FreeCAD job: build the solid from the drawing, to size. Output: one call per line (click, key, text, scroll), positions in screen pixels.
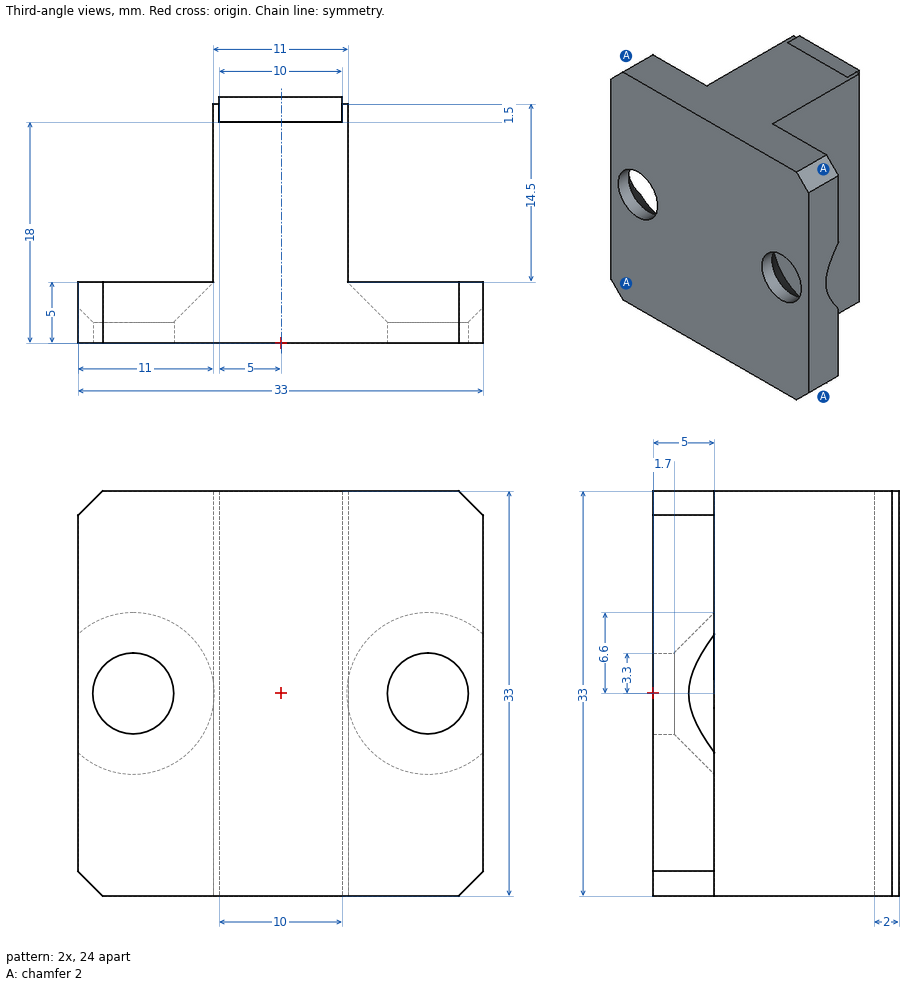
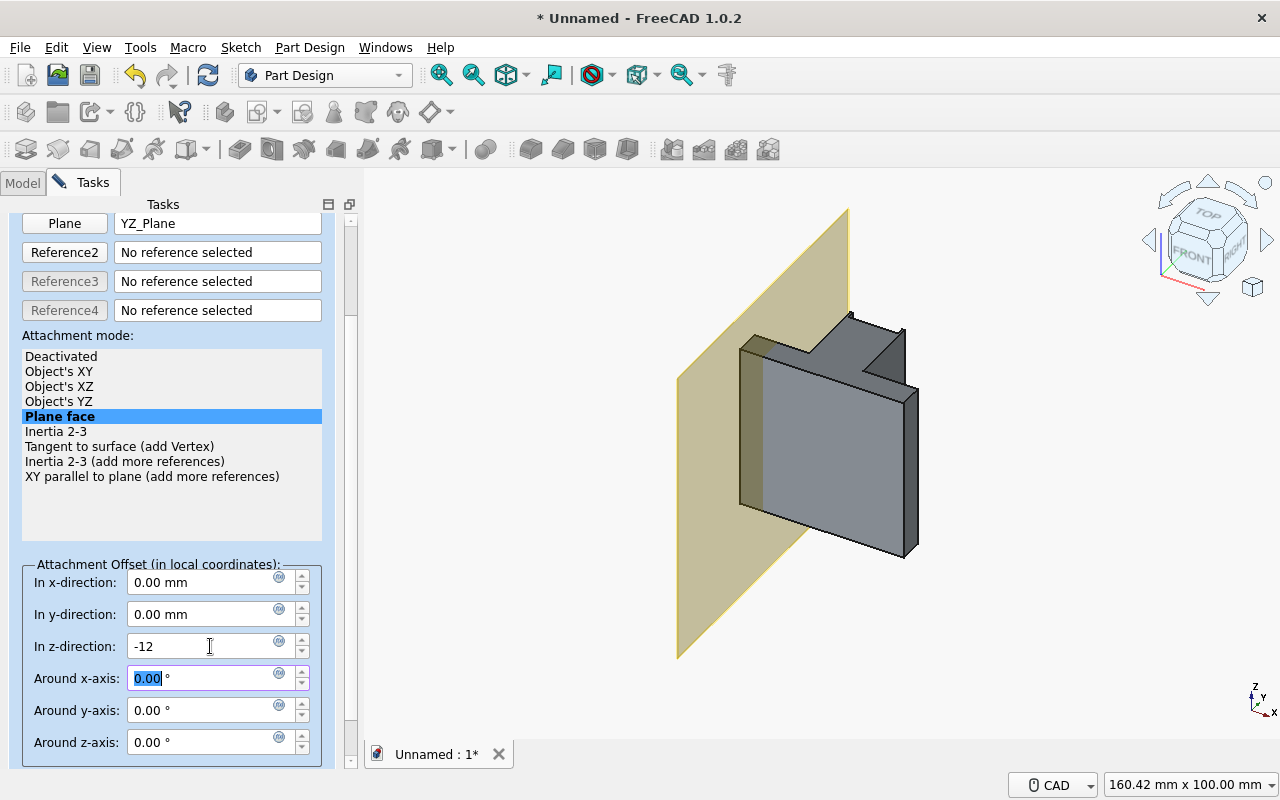
scroll(351, 491, up, 3)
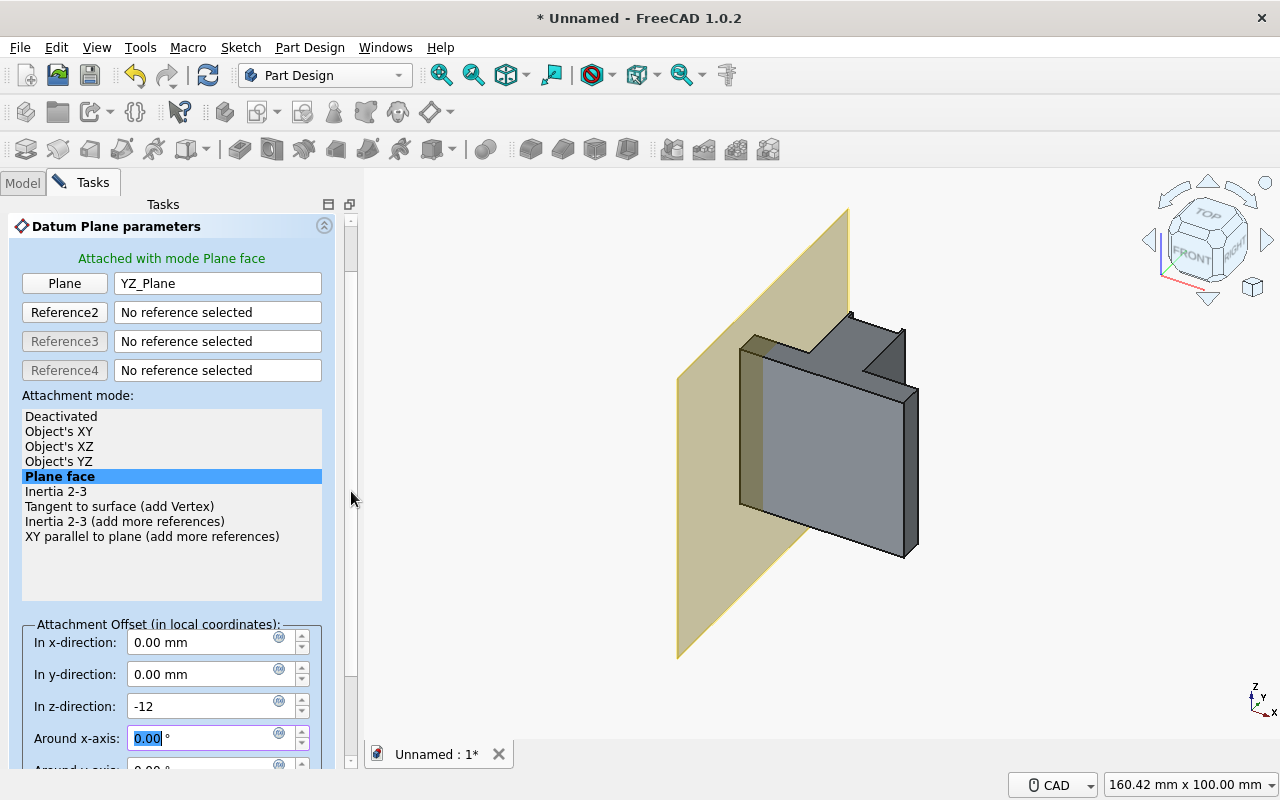
click(124, 243)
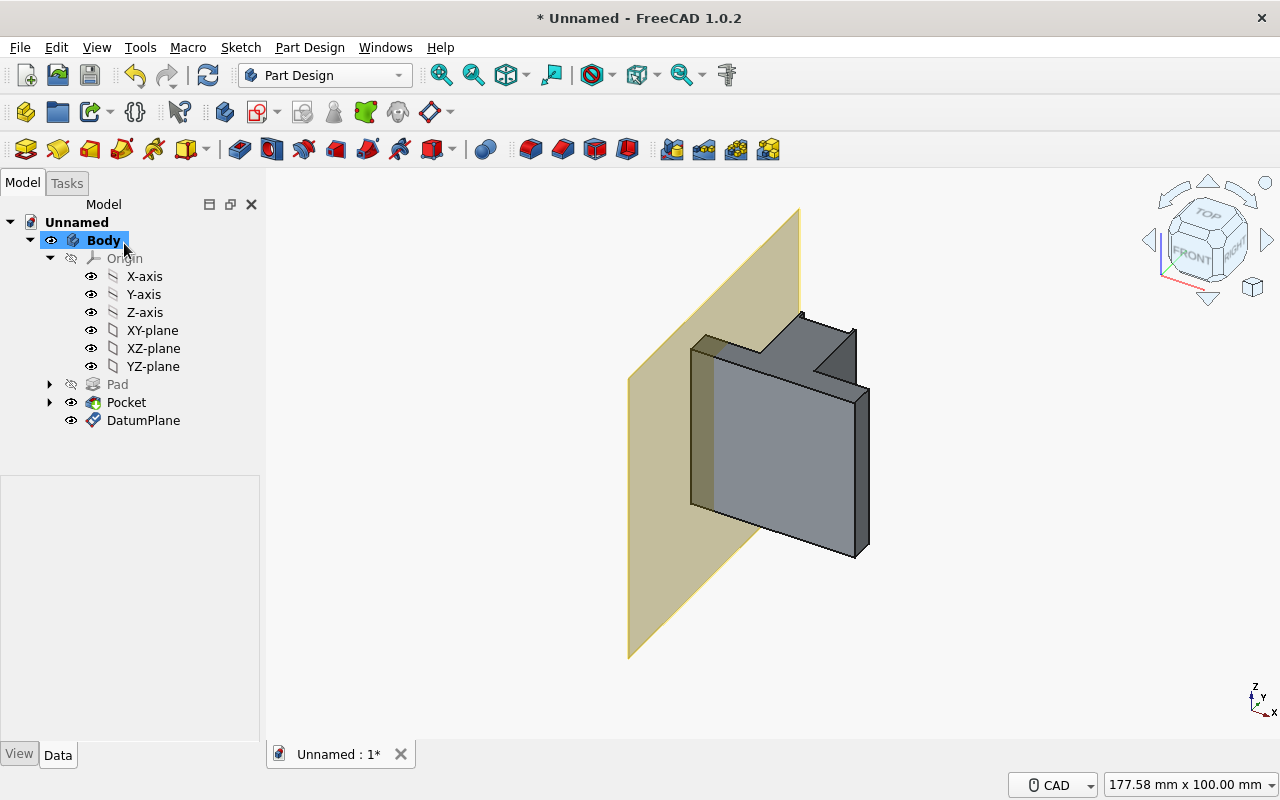
click(116, 420)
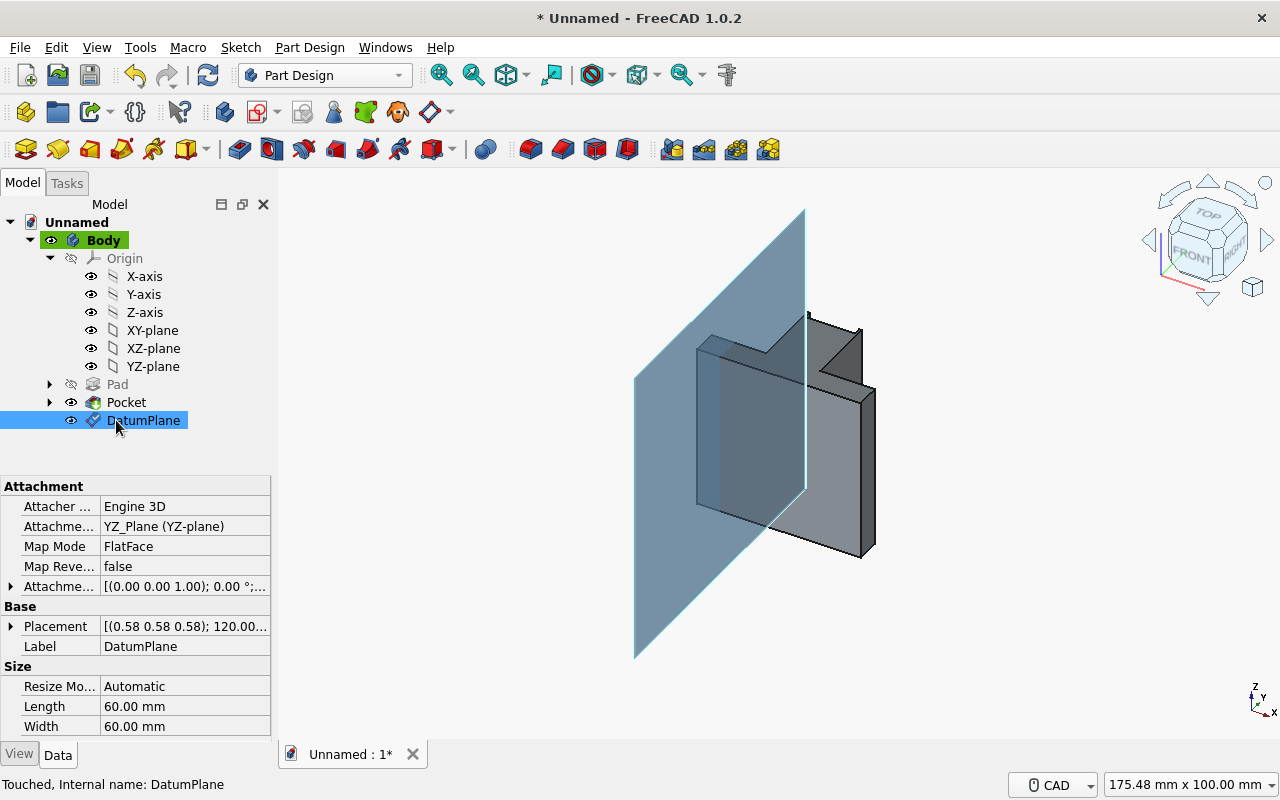
click(258, 112)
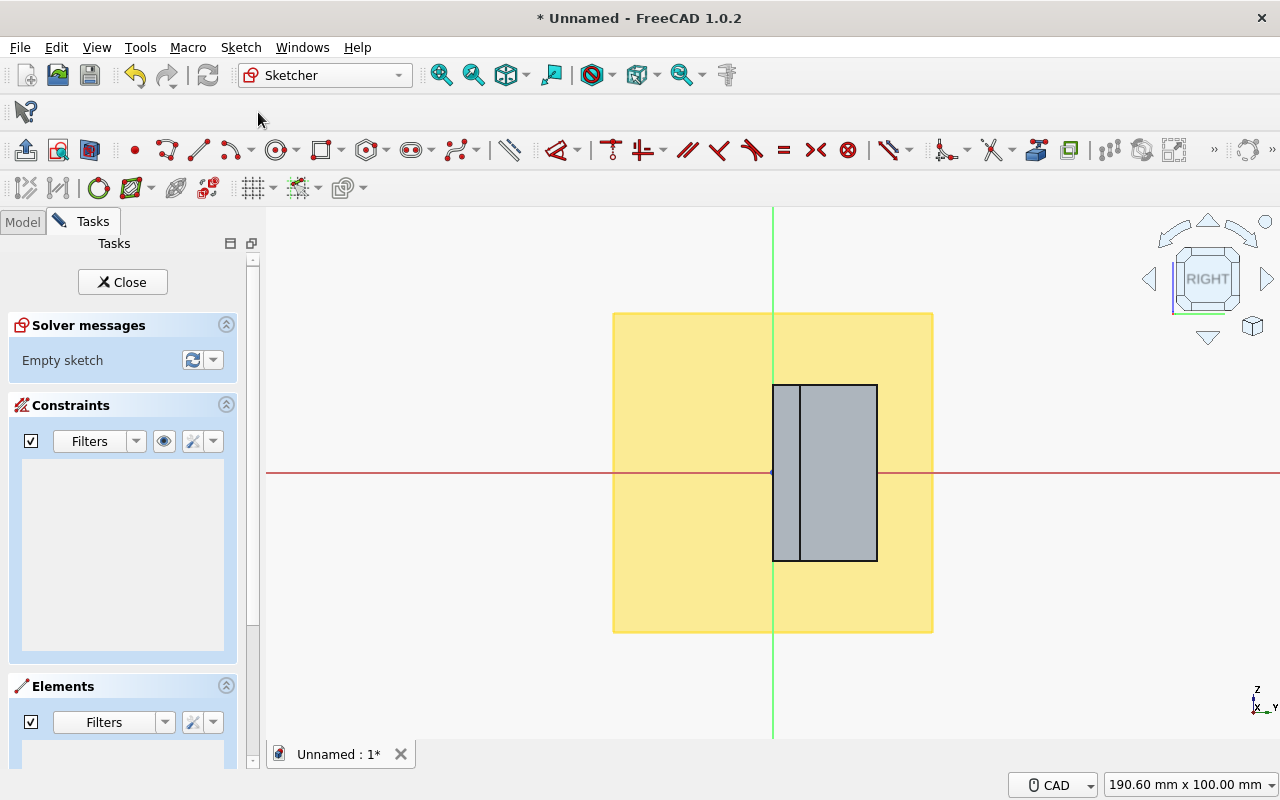
key(q)
key(s)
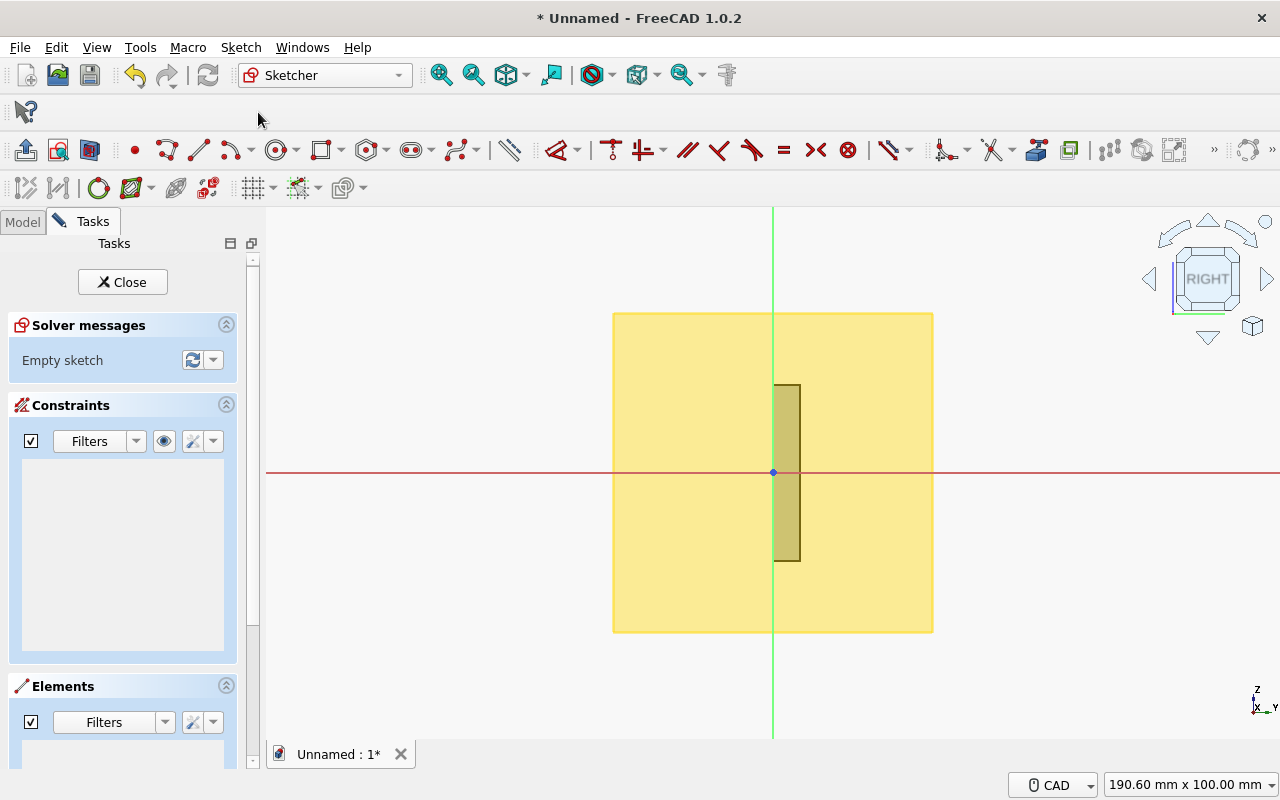
scroll(796, 453, up, 11)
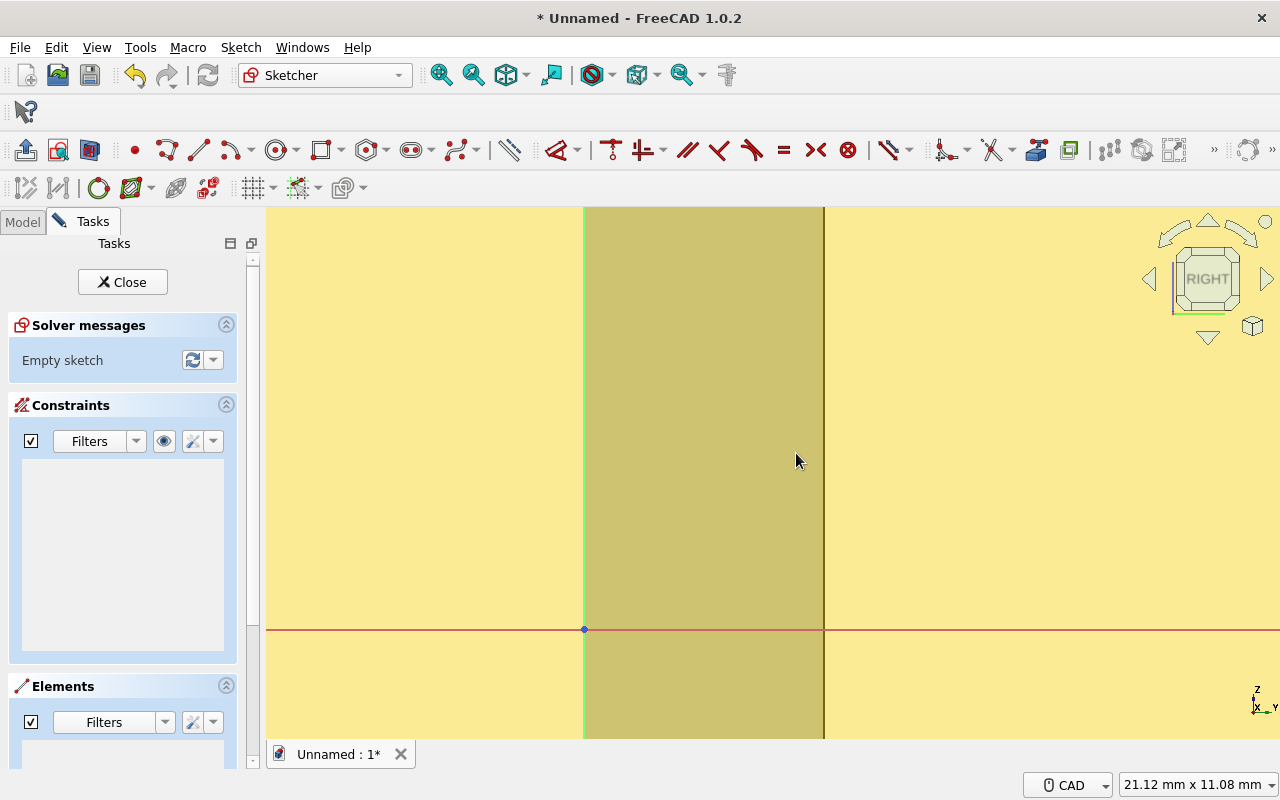
click(168, 150)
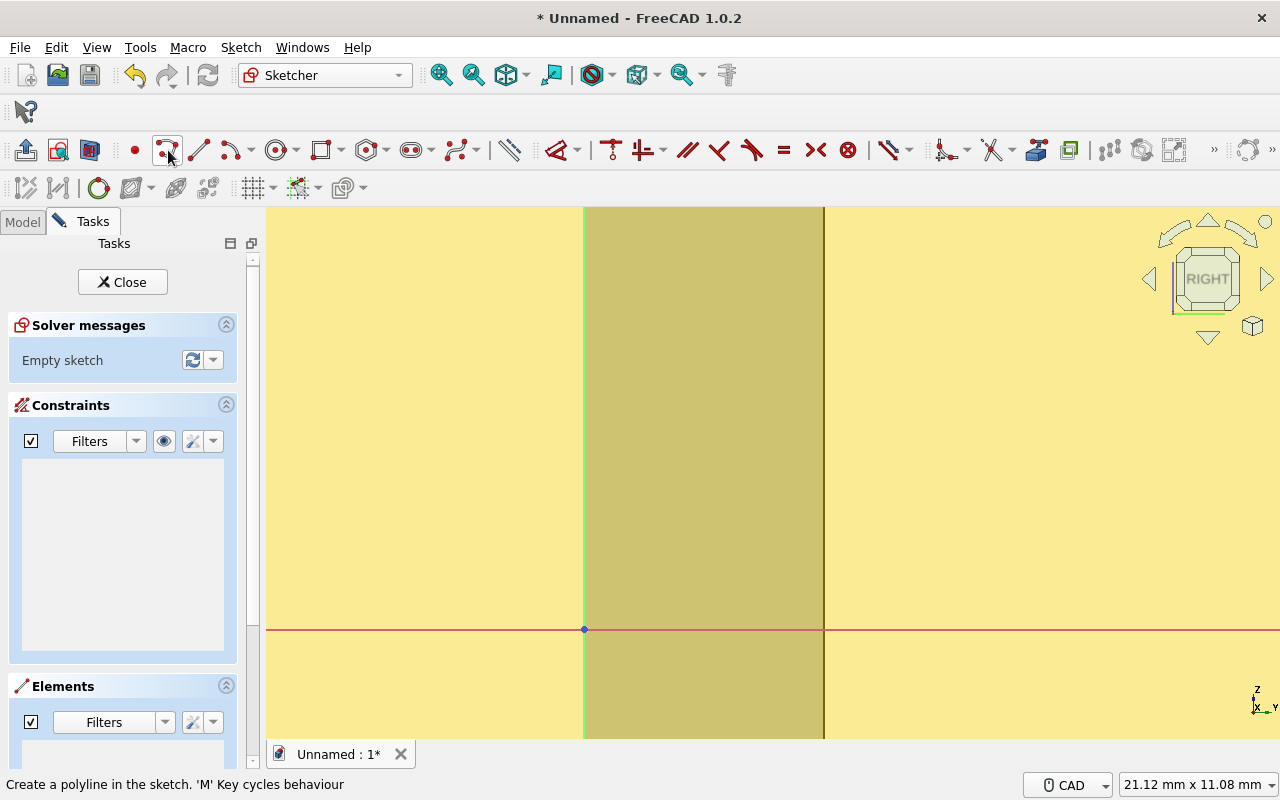
click(584, 630)
click(824, 621)
click(824, 313)
click(666, 471)
click(593, 471)
click(584, 630)
key(Escape)
key(Escape)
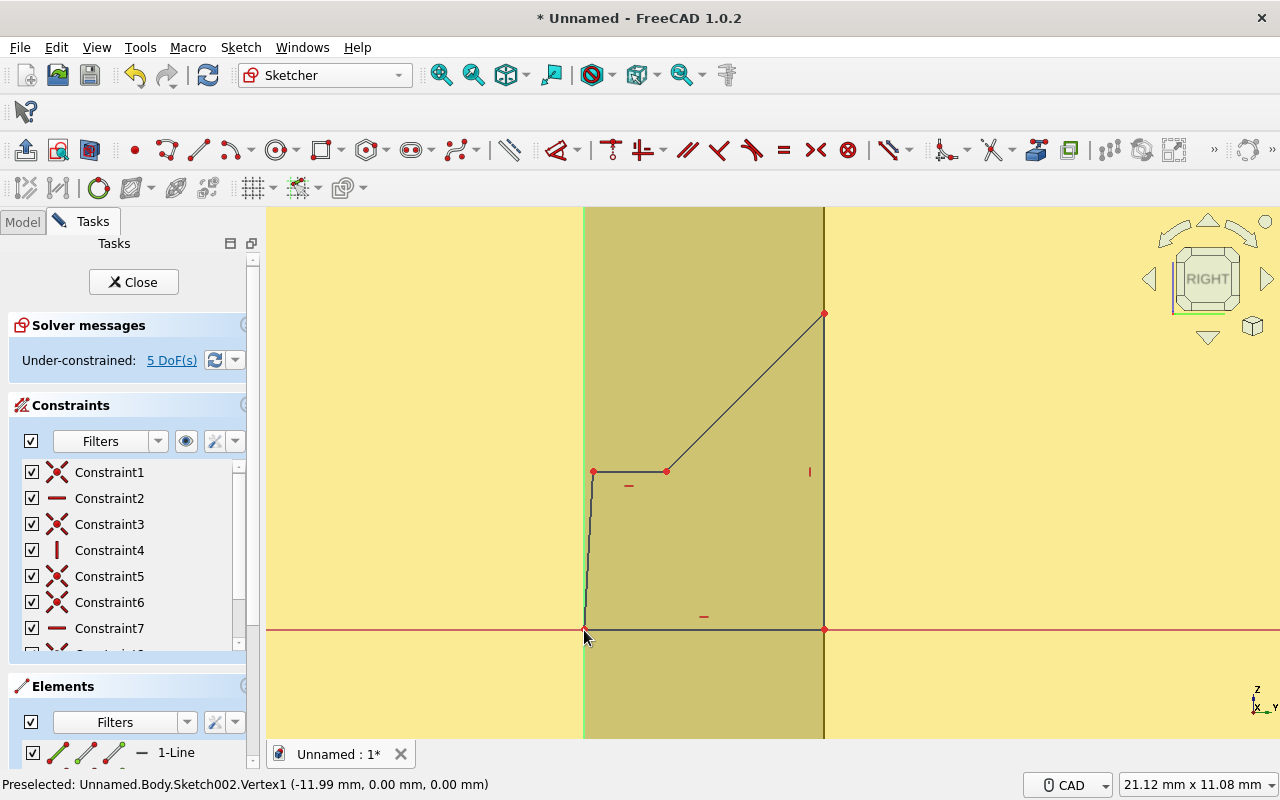
click(587, 582)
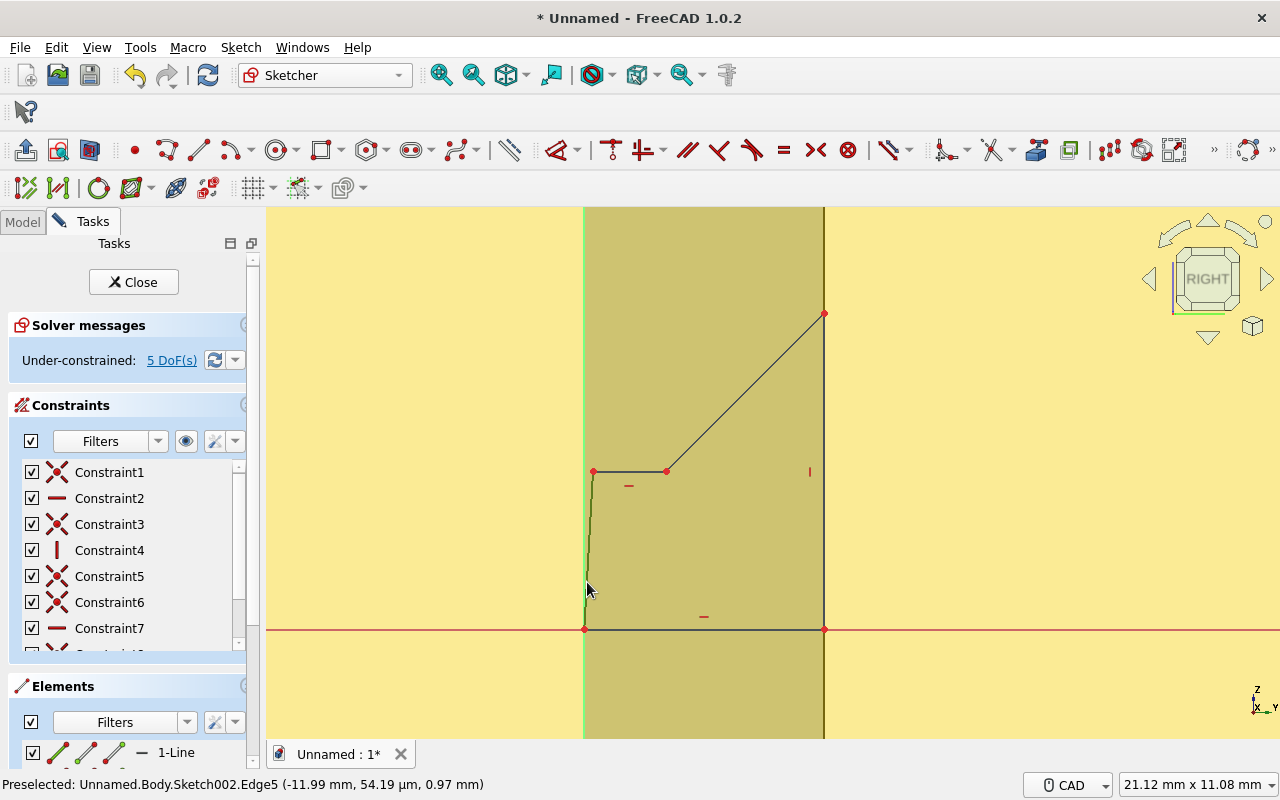
click(666, 150)